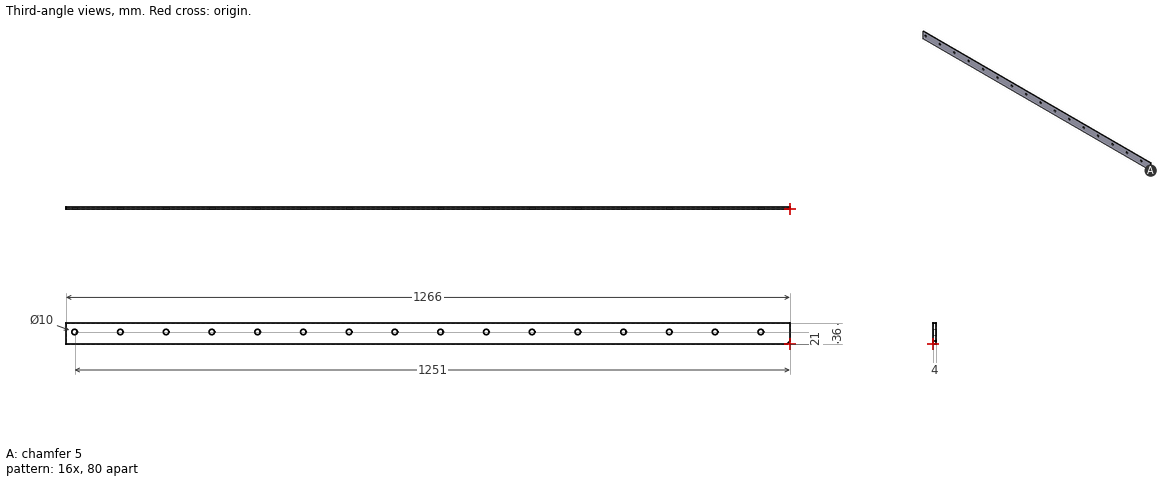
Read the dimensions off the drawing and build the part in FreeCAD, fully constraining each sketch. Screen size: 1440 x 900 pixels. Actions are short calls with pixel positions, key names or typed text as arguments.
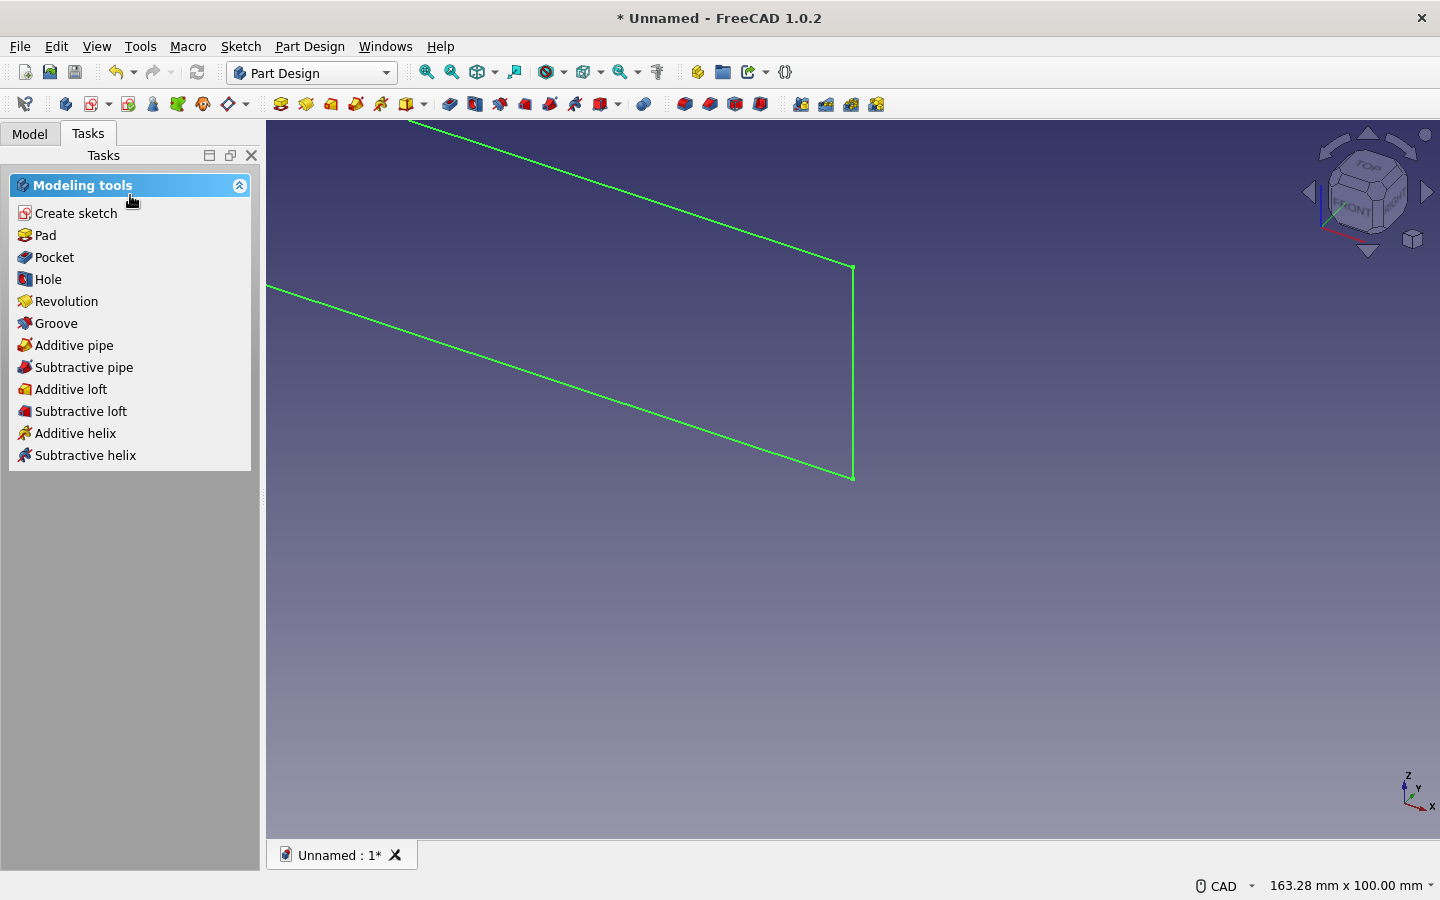
click(281, 104)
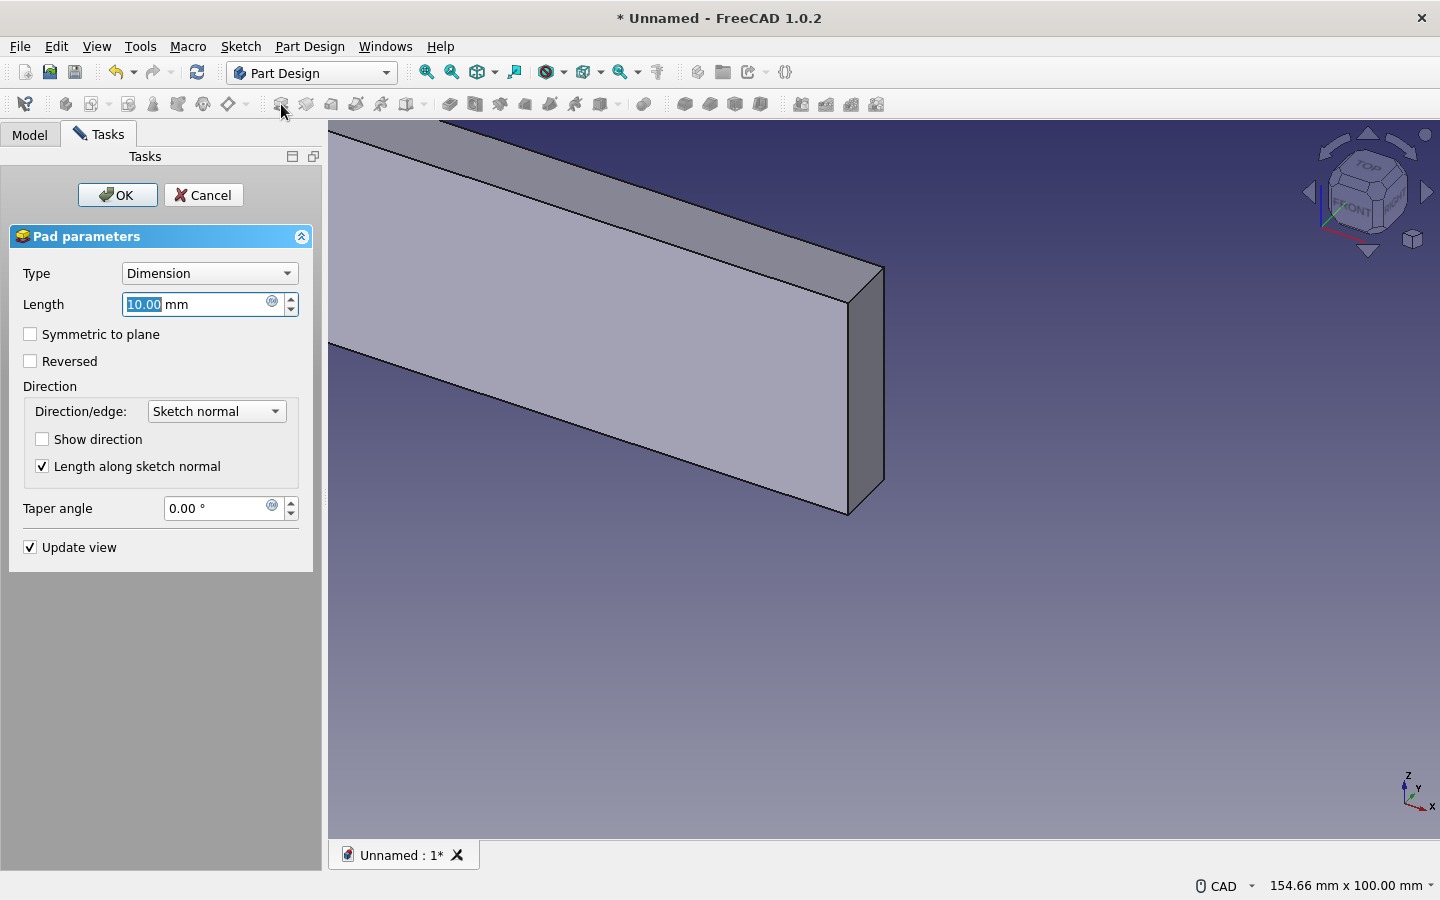
text(4)
key(Tab)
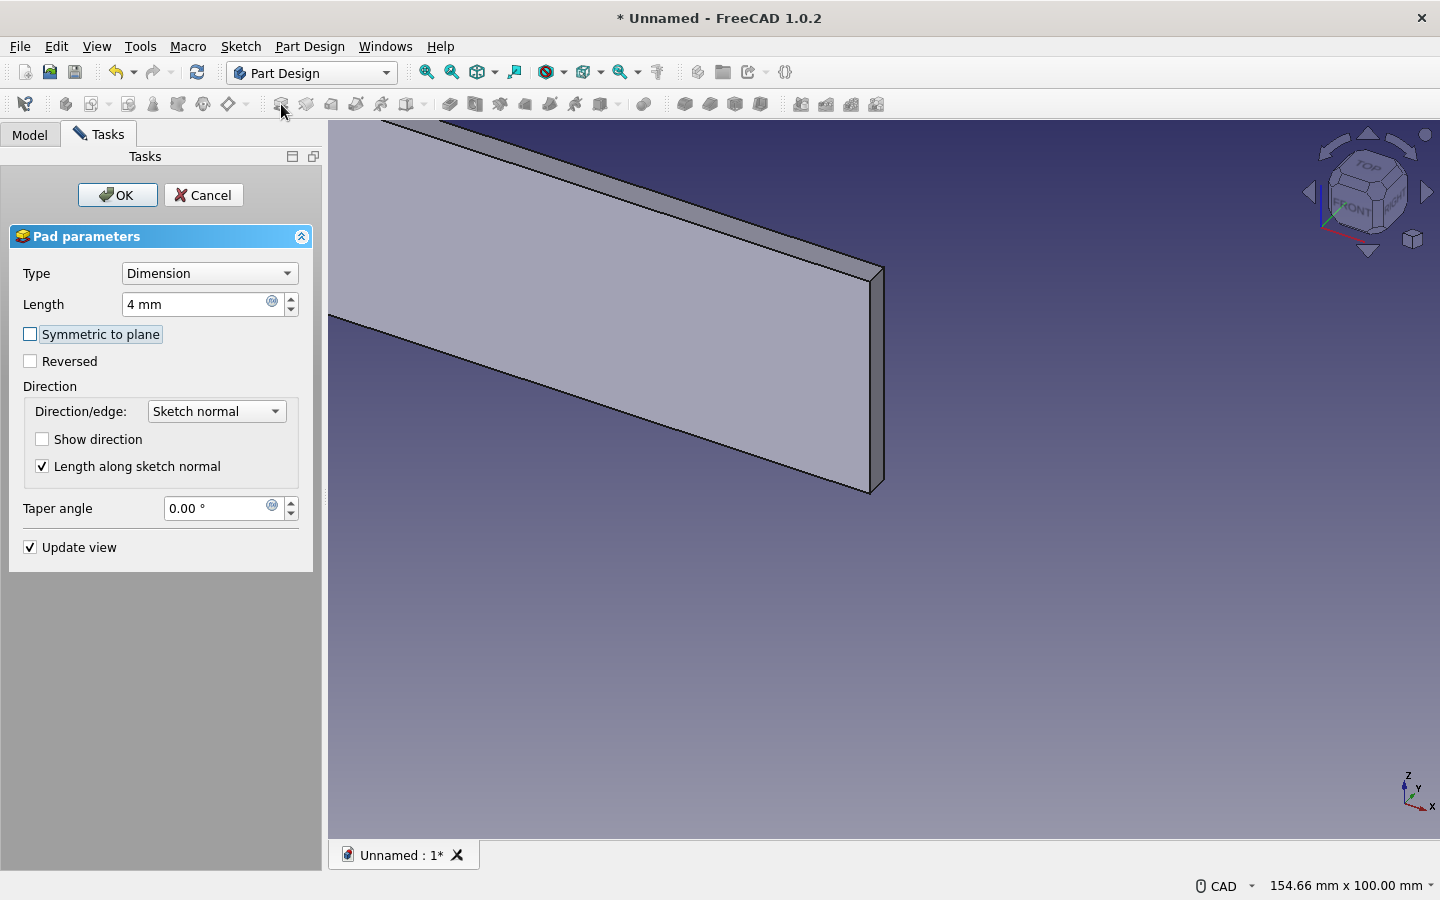
click(31, 361)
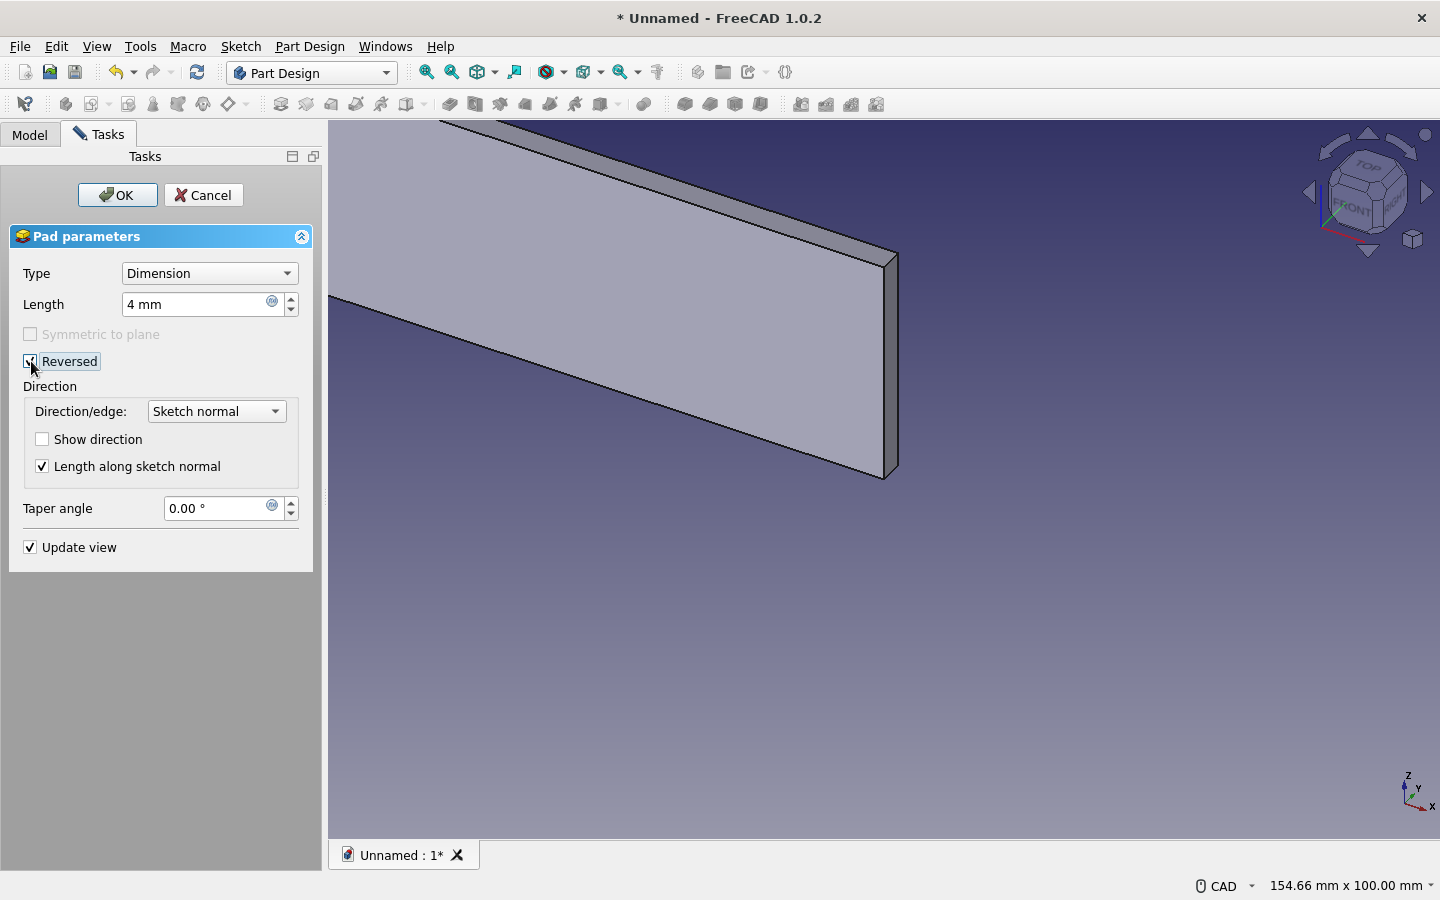
click(118, 195)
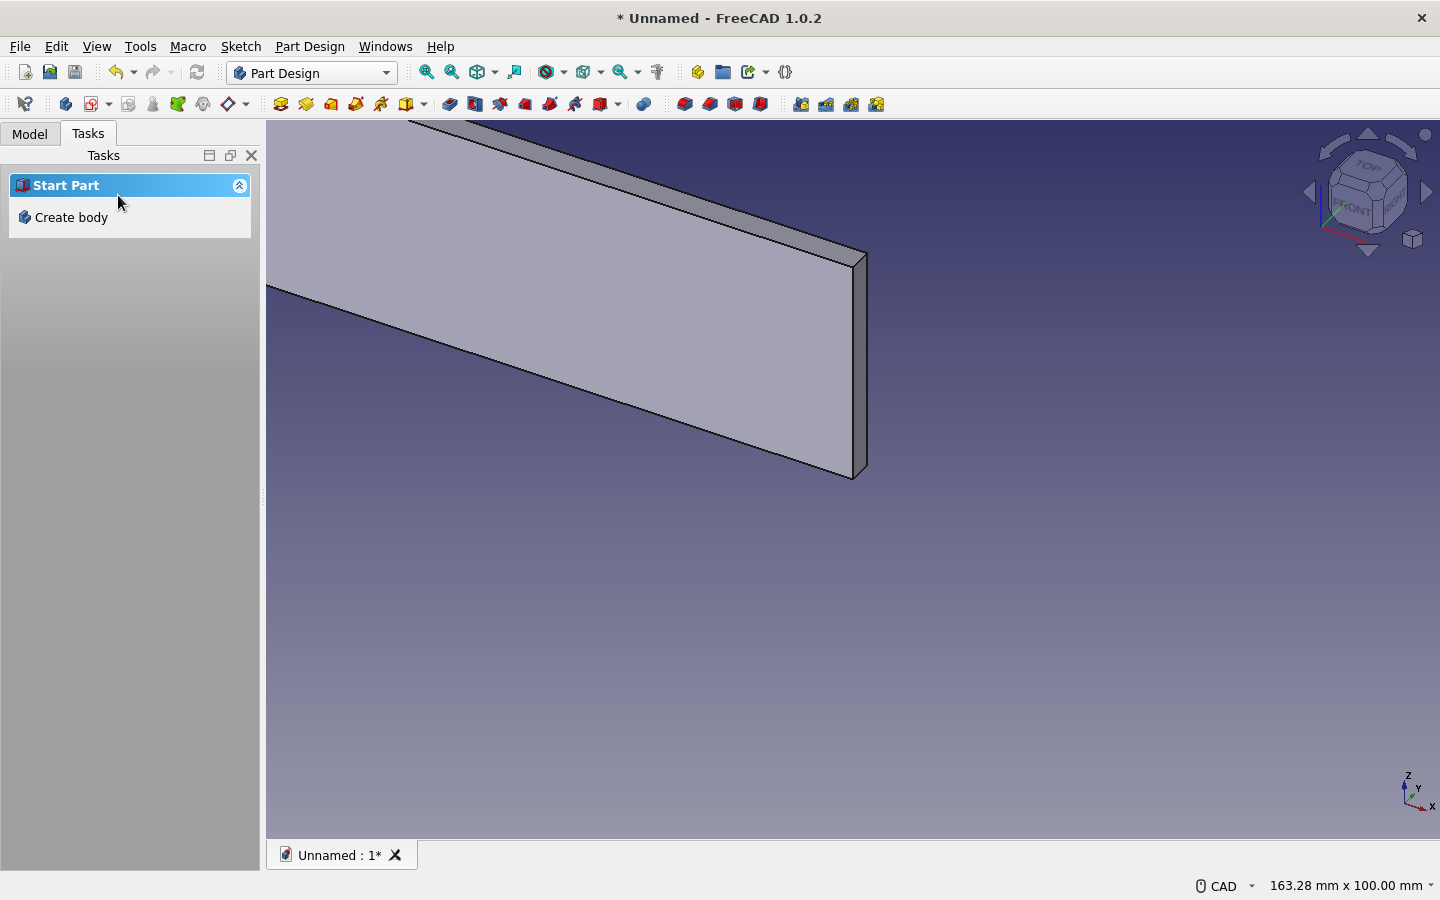
click(427, 72)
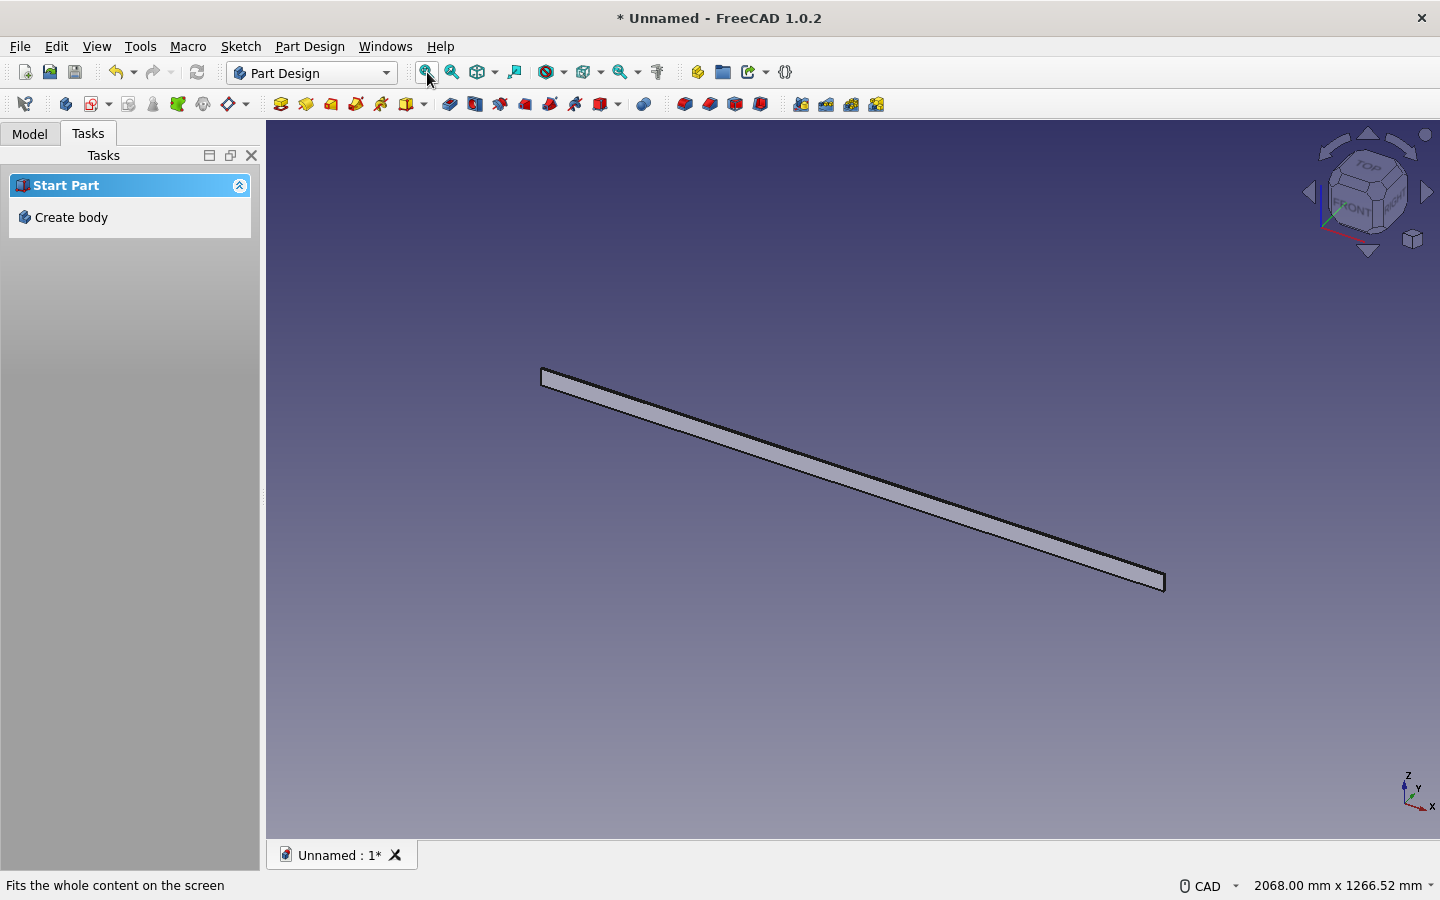
scroll(1164, 590, up, 15)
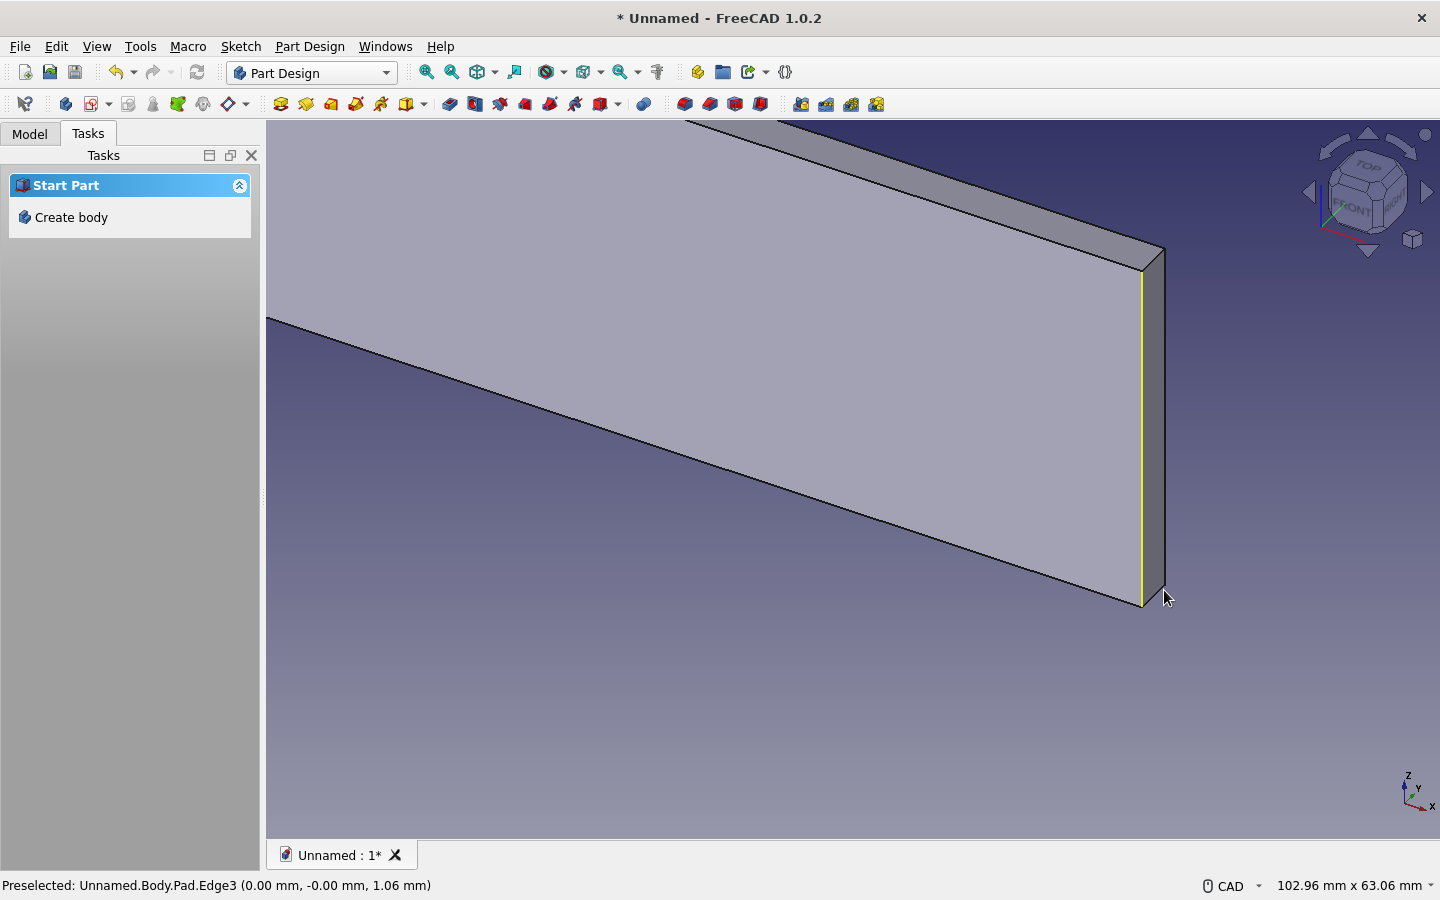
click(427, 72)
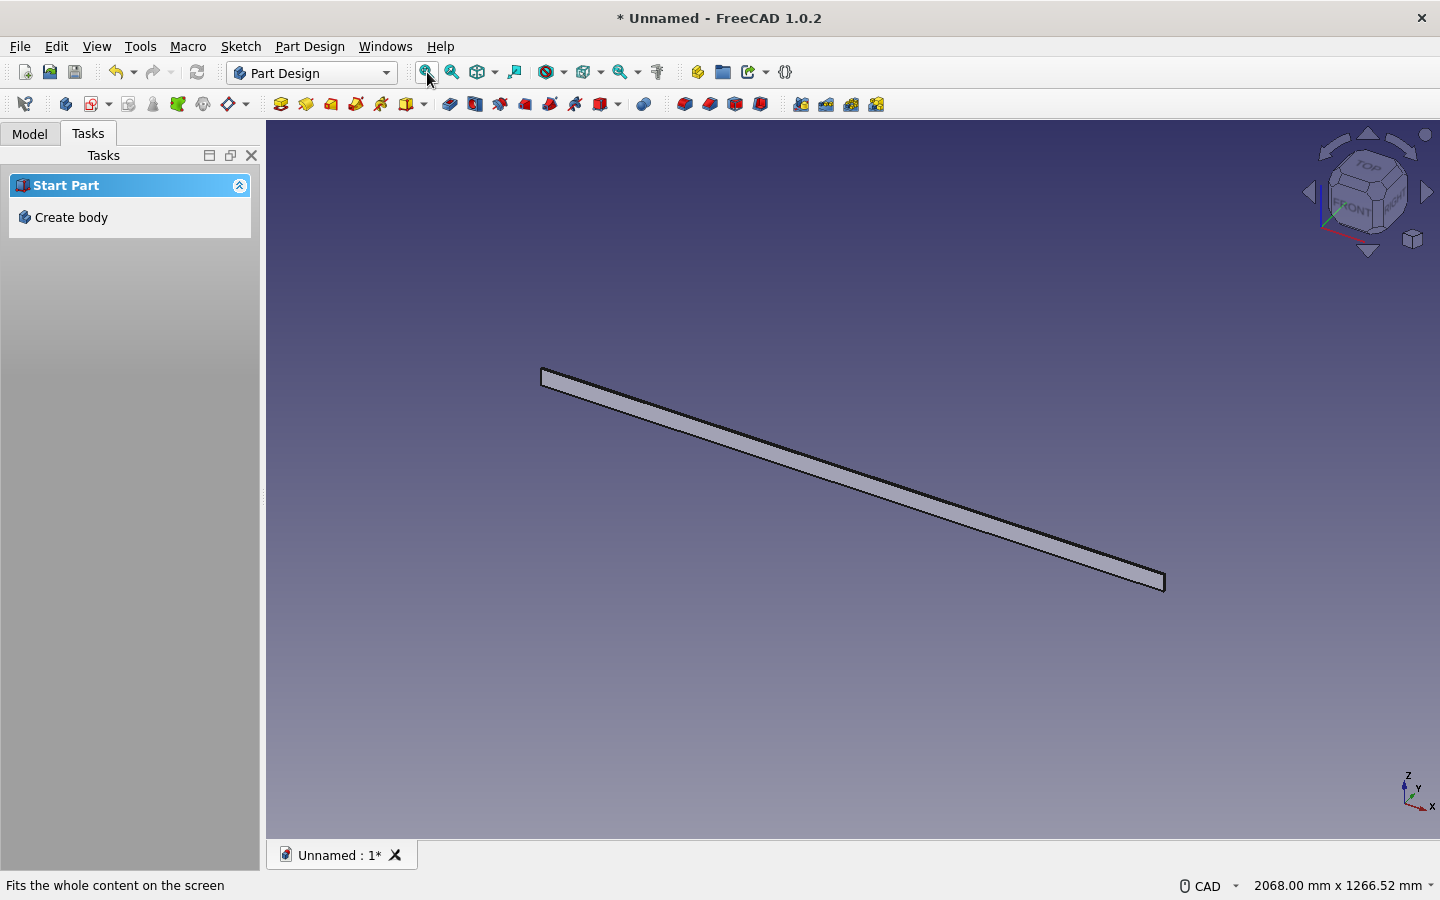
key(0)